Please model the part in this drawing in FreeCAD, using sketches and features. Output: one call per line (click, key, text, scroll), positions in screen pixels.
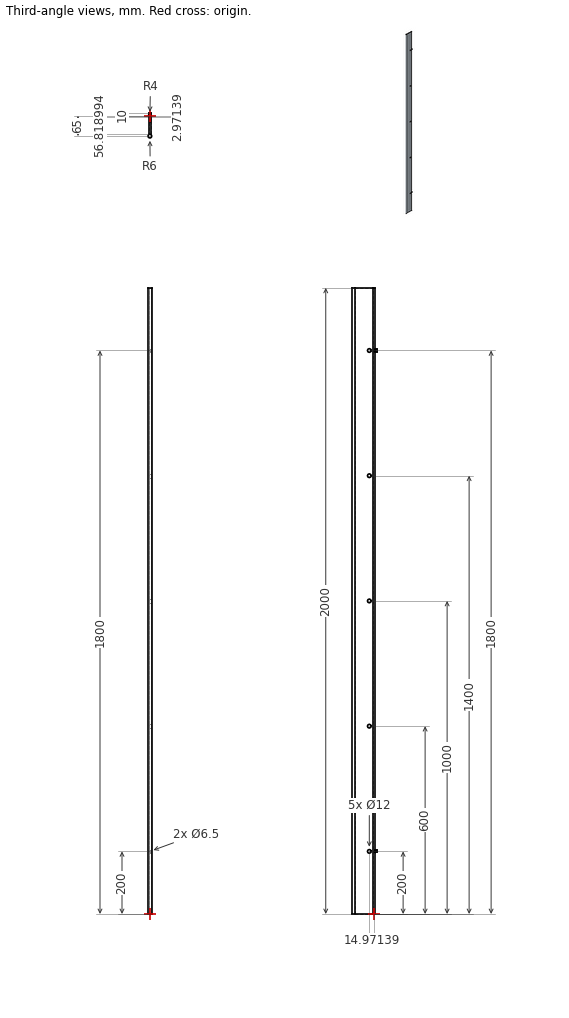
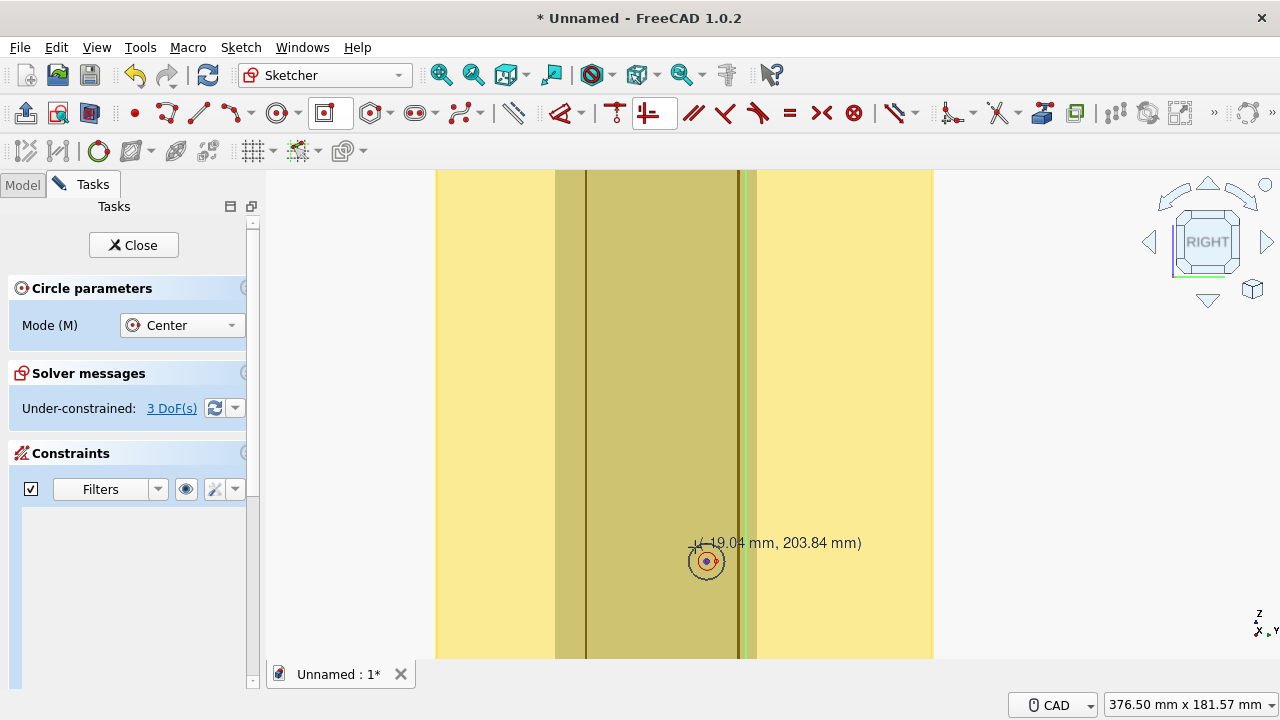
scroll(704, 528, down, 14)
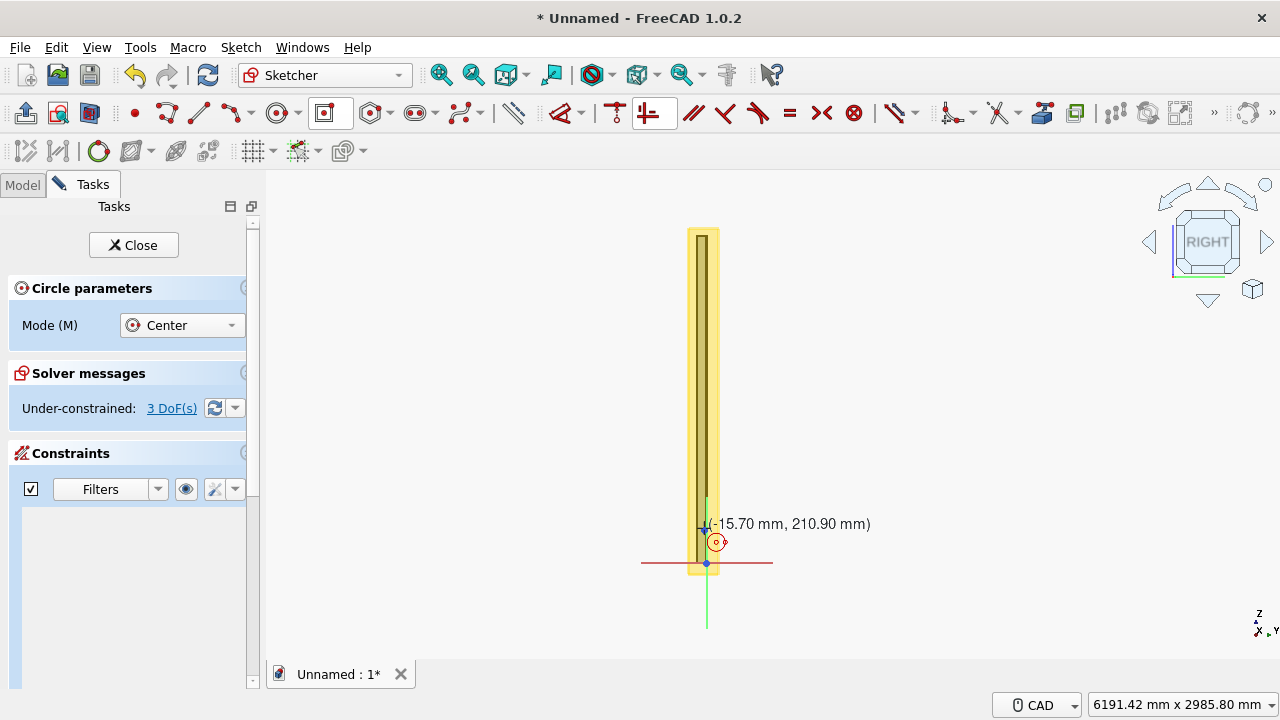
scroll(705, 465, up, 16)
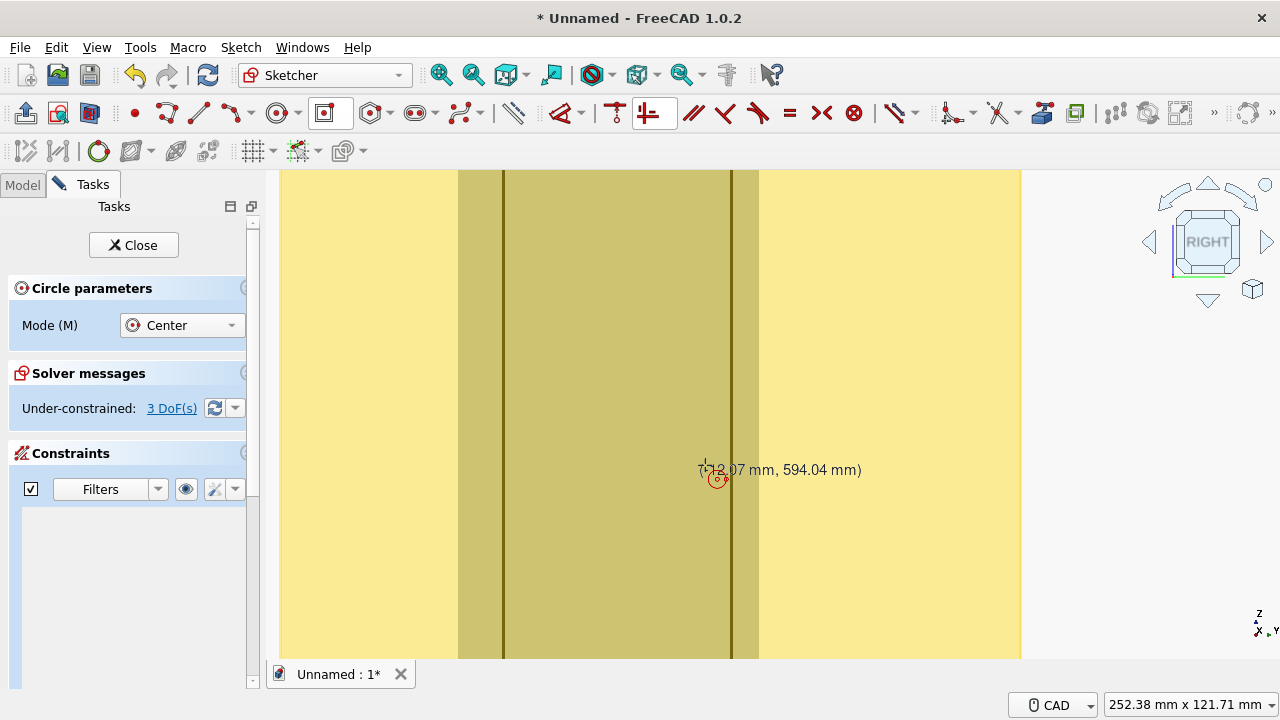
scroll(705, 476, down, 15)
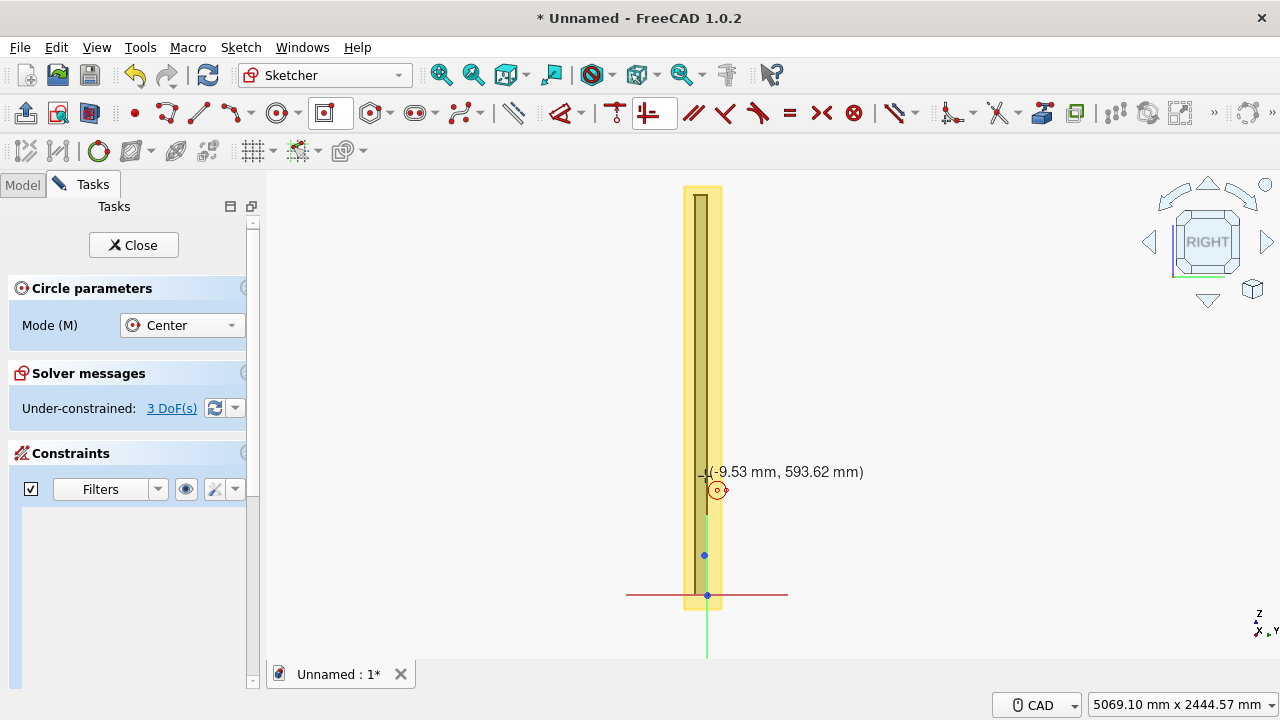
scroll(704, 475, up, 9)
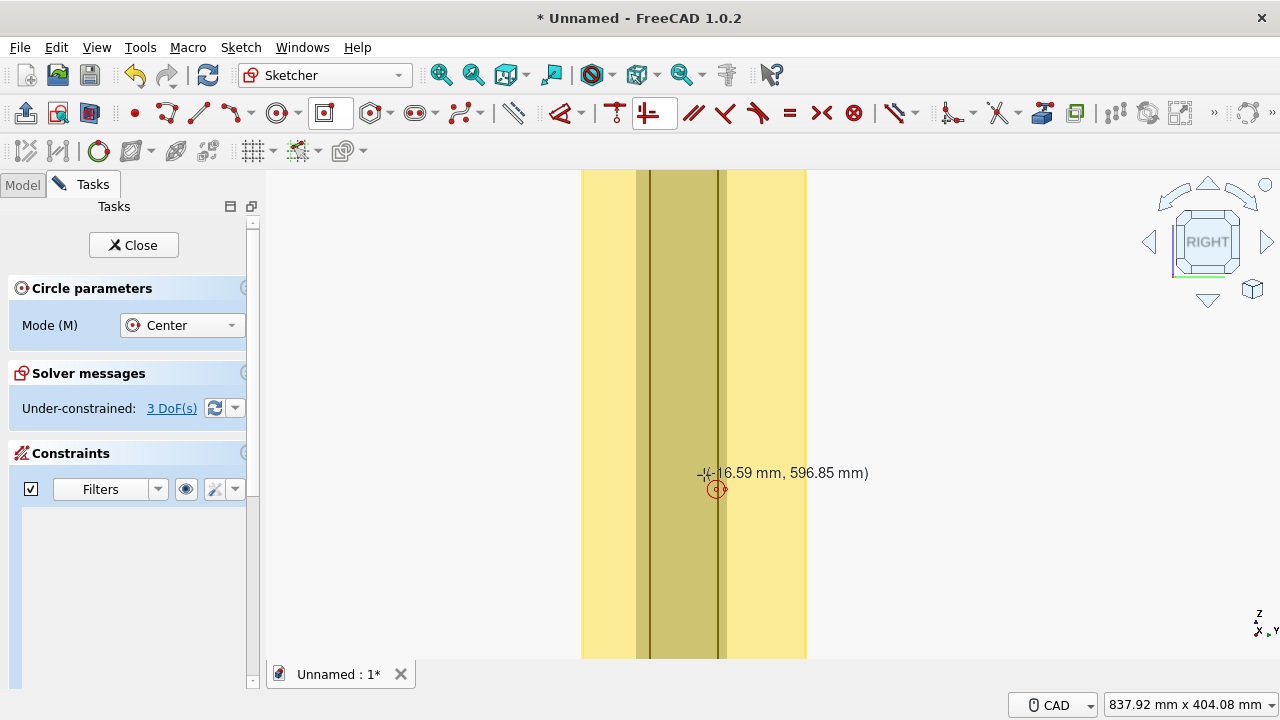
click(704, 474)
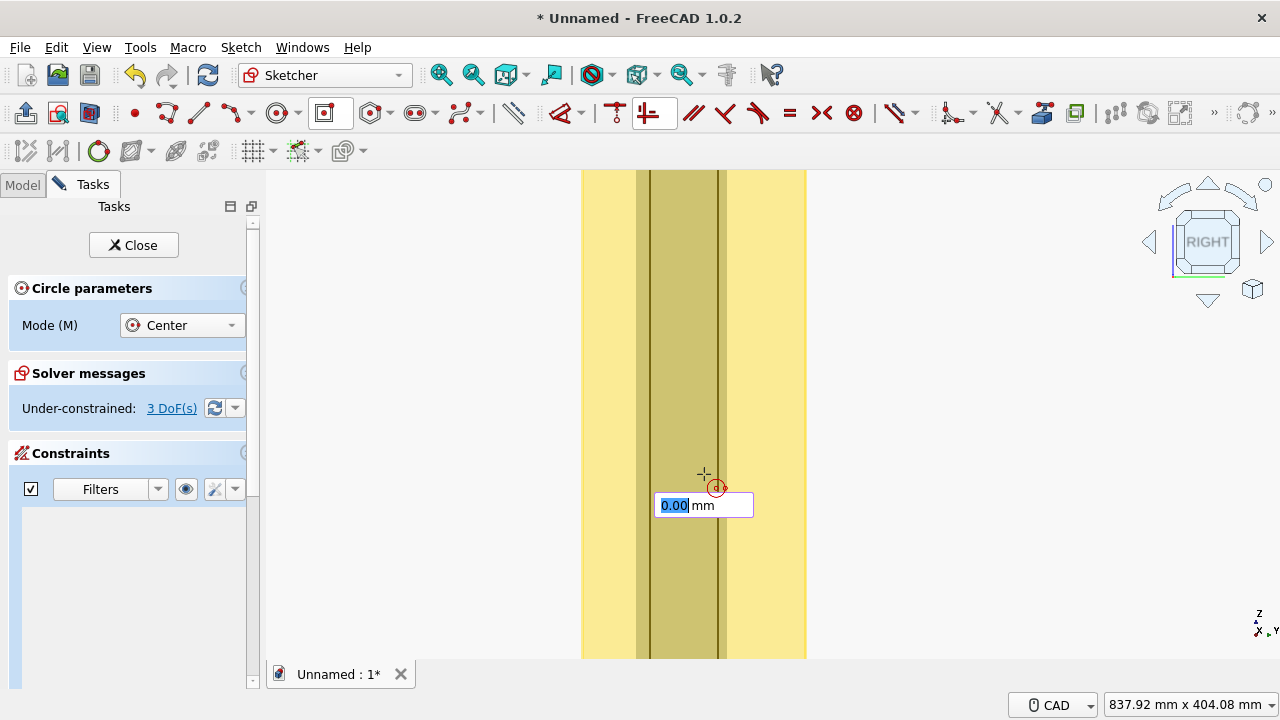
scroll(699, 469, up, 4)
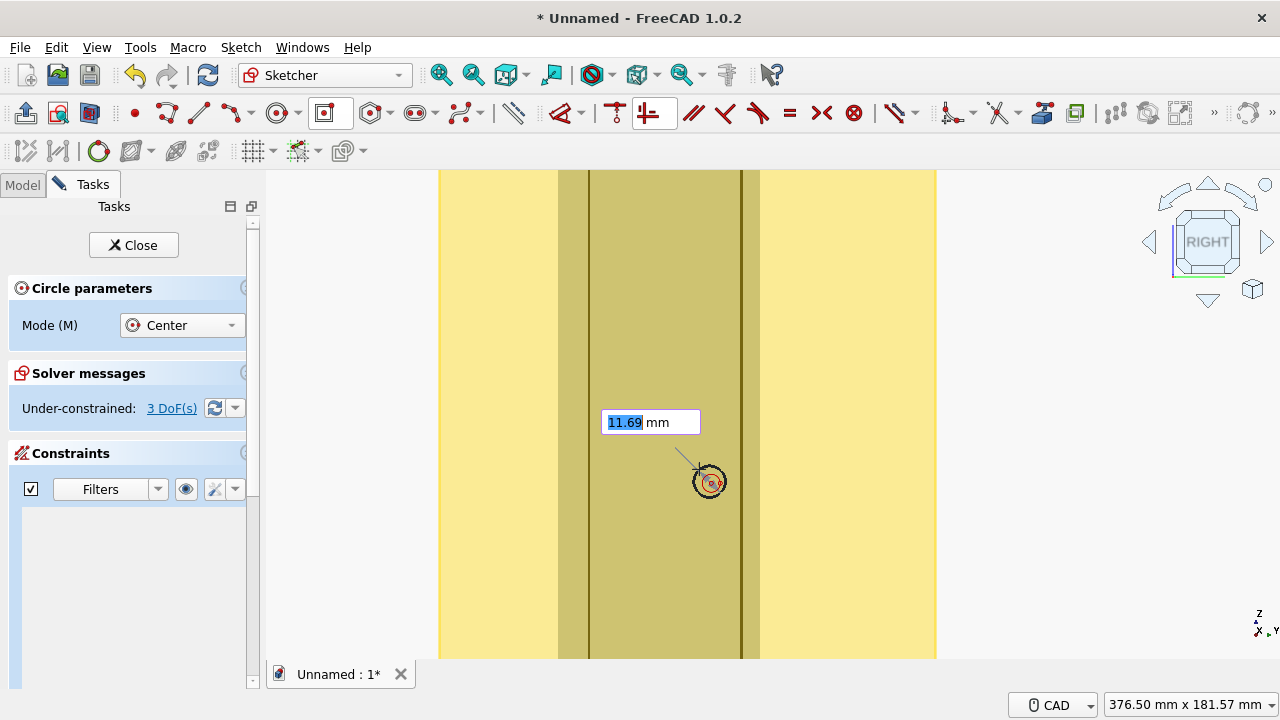
click(698, 468)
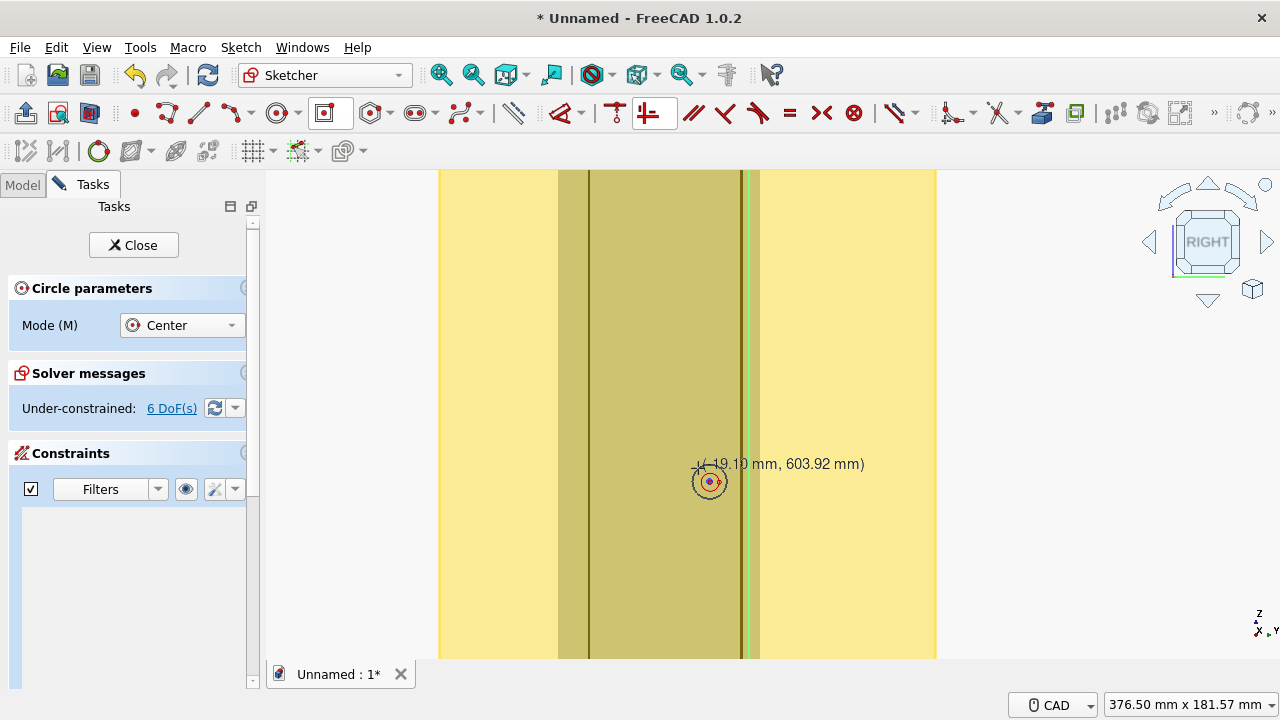
scroll(703, 463, down, 14)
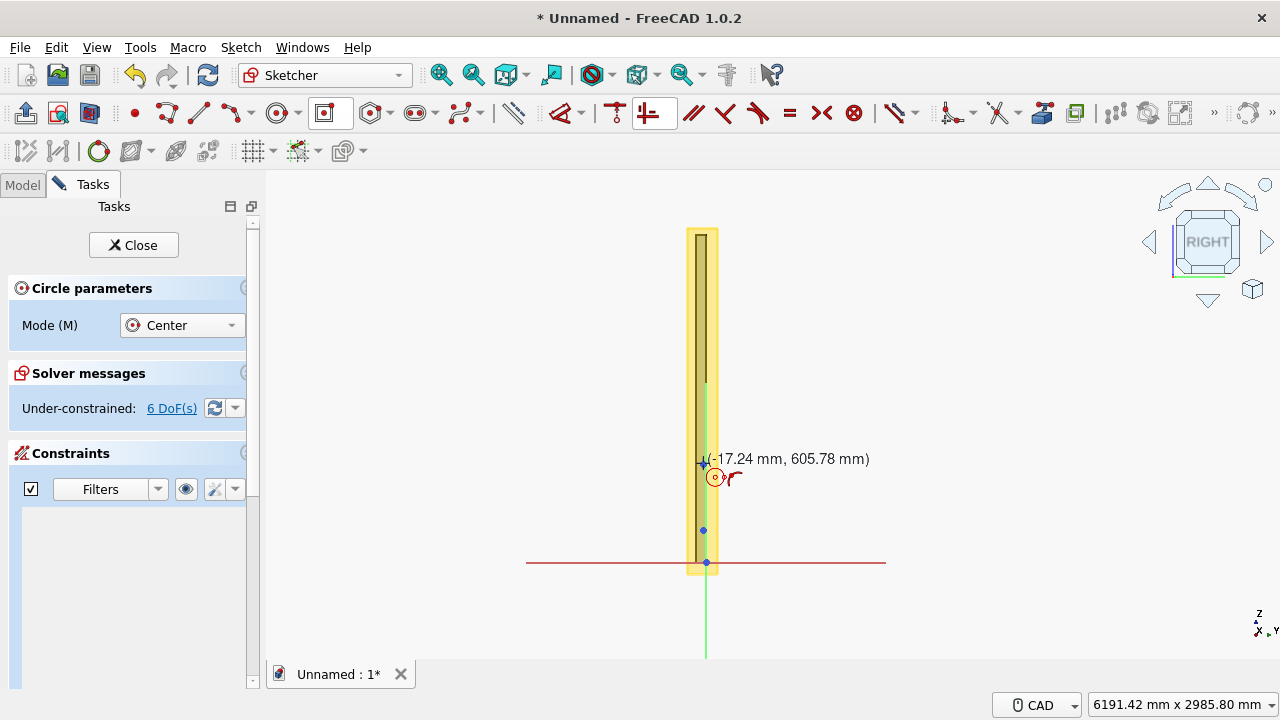
scroll(704, 399, up, 16)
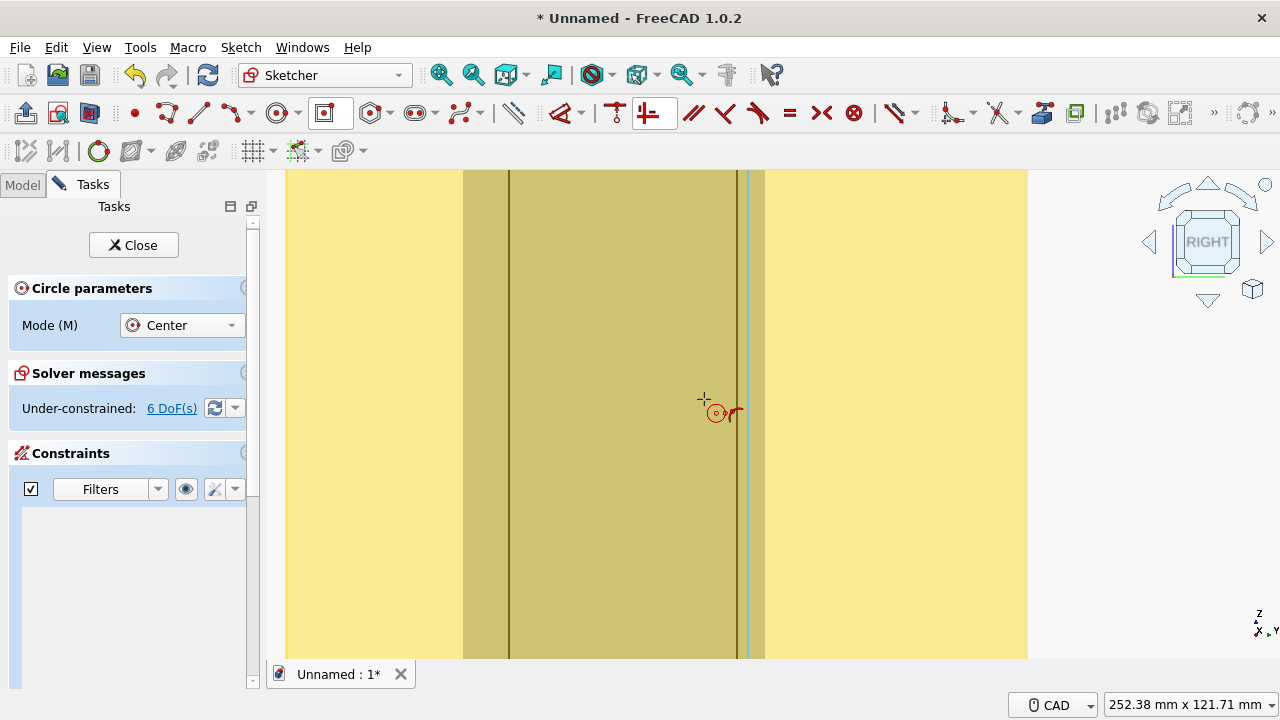
scroll(704, 395, down, 15)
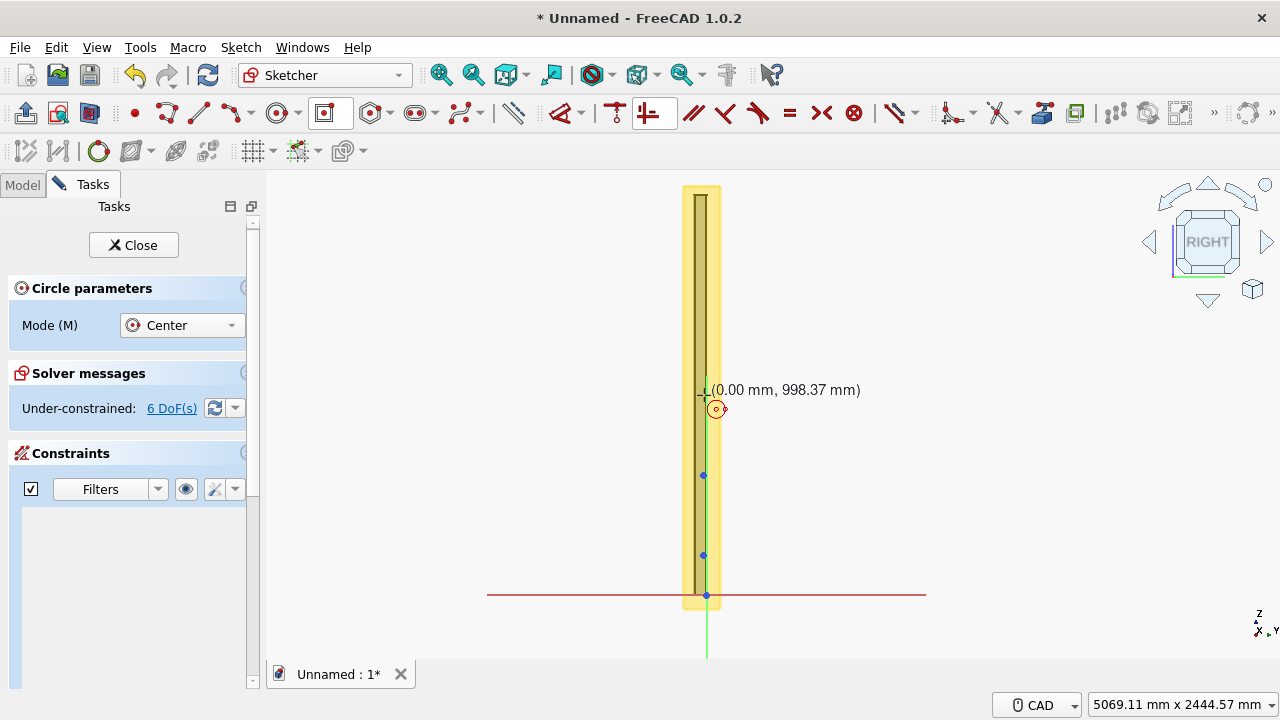
scroll(704, 395, up, 9)